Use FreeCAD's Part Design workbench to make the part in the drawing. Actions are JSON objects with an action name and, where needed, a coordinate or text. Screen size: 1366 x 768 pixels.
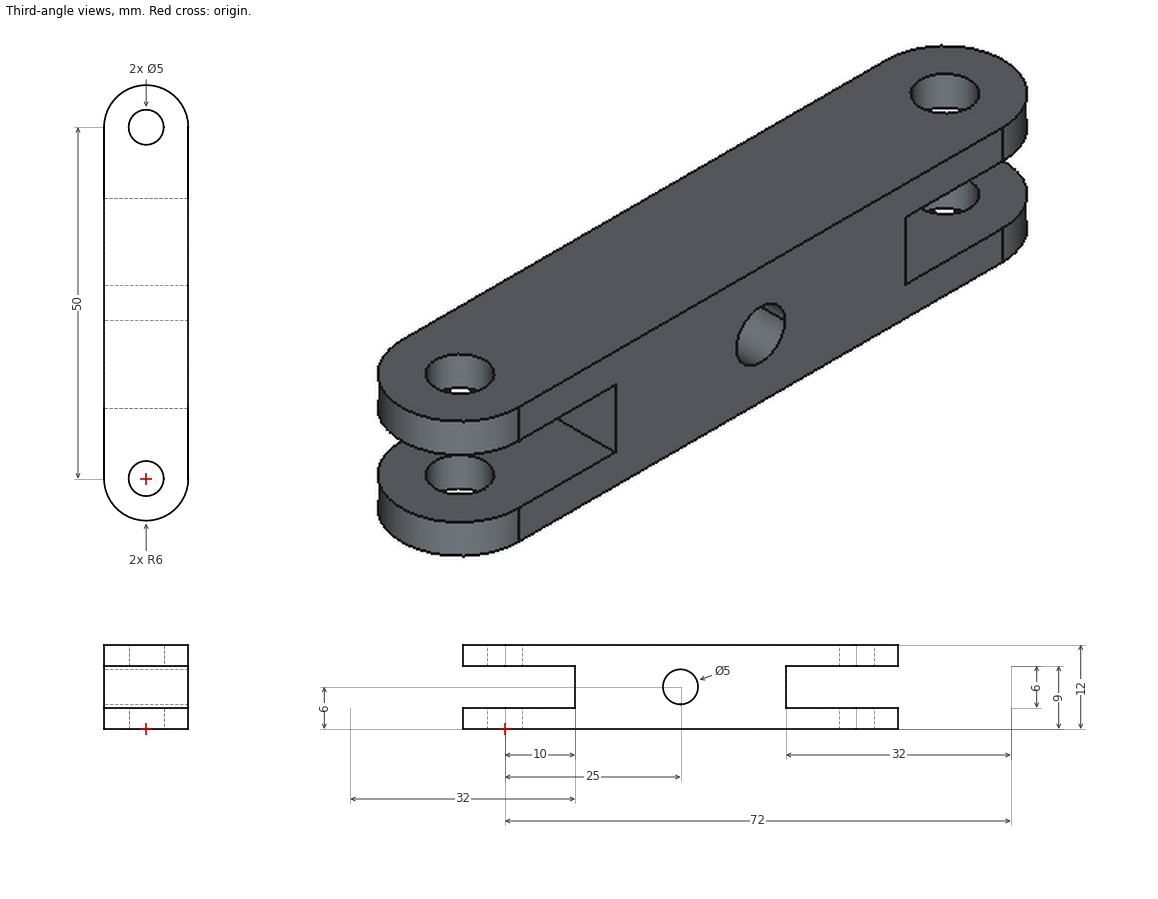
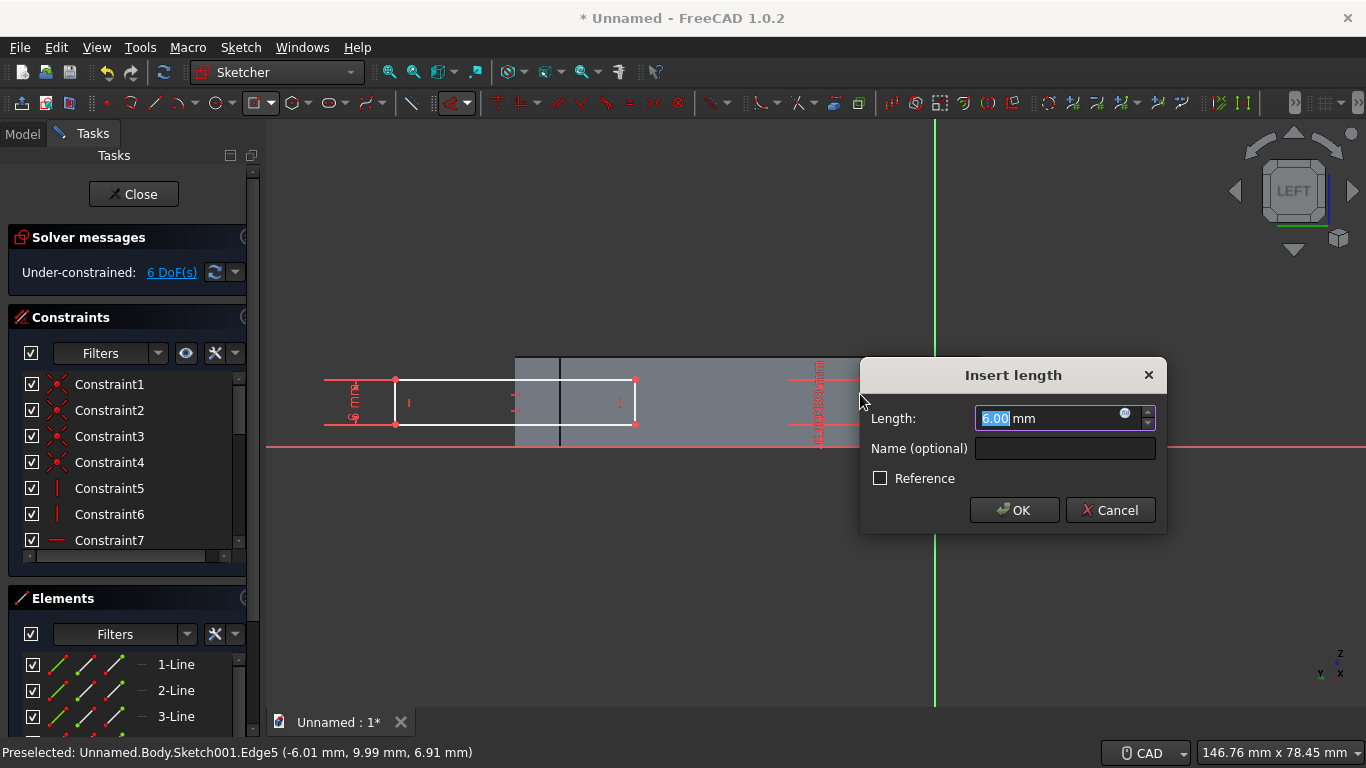
{"action": "type", "text": "6"}
{"action": "key", "text": "Return"}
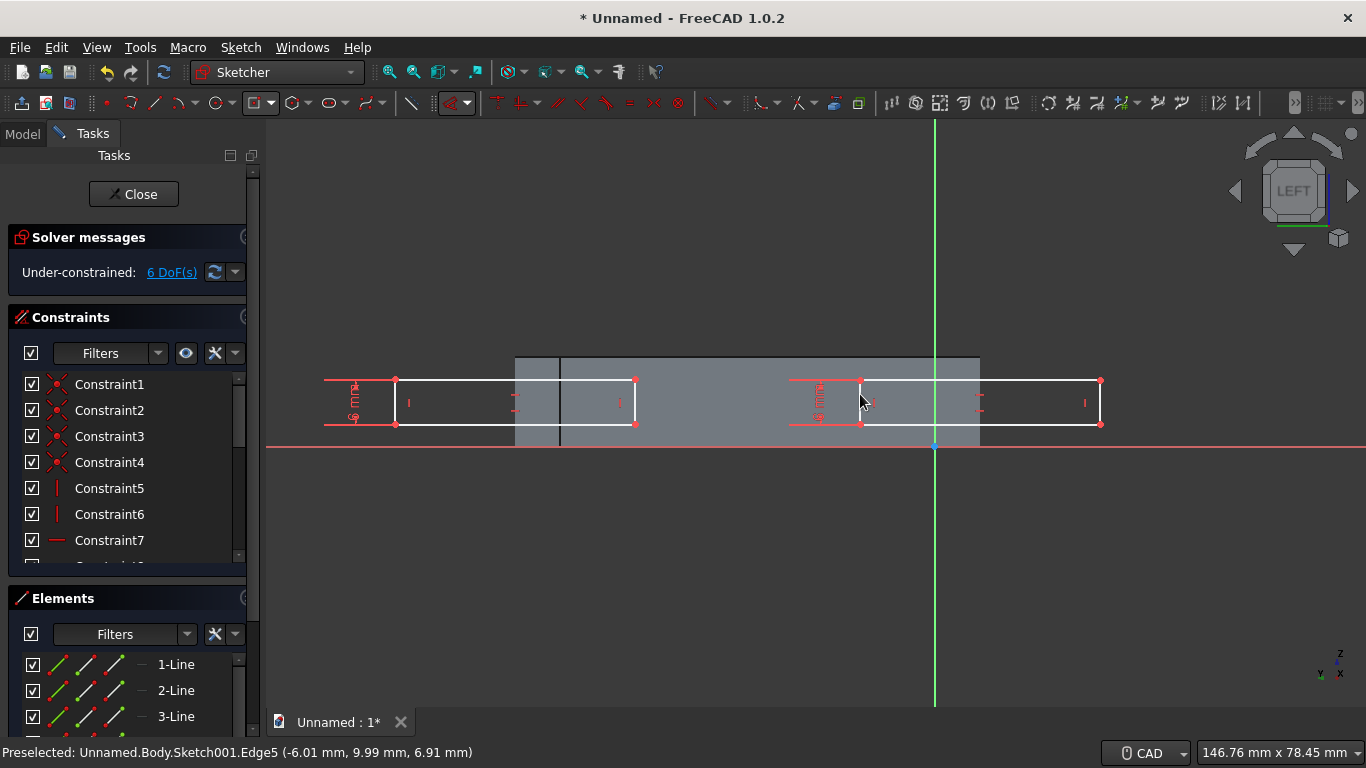
{"action": "left_click", "coordinate": [467, 425]}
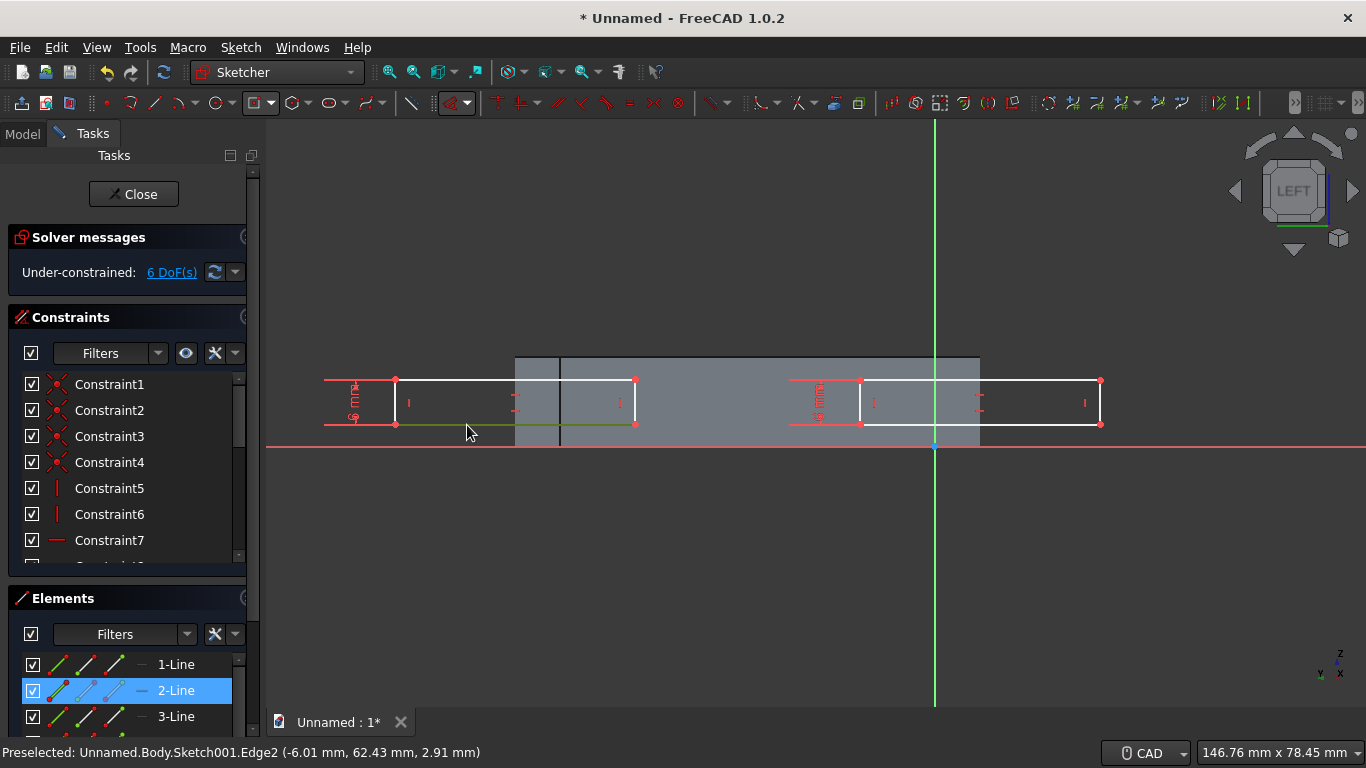
{"action": "key", "text": "l"}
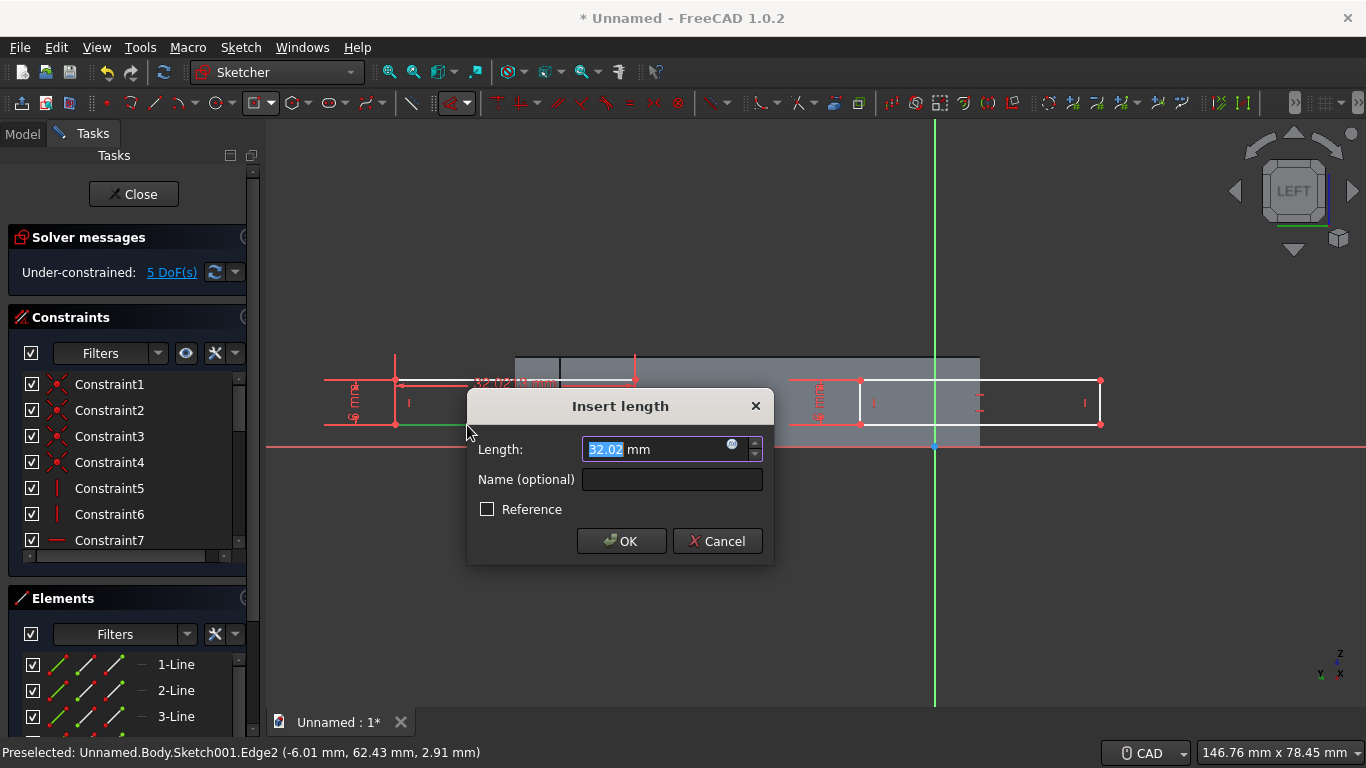
{"action": "type", "text": "32"}
{"action": "key", "text": "Return"}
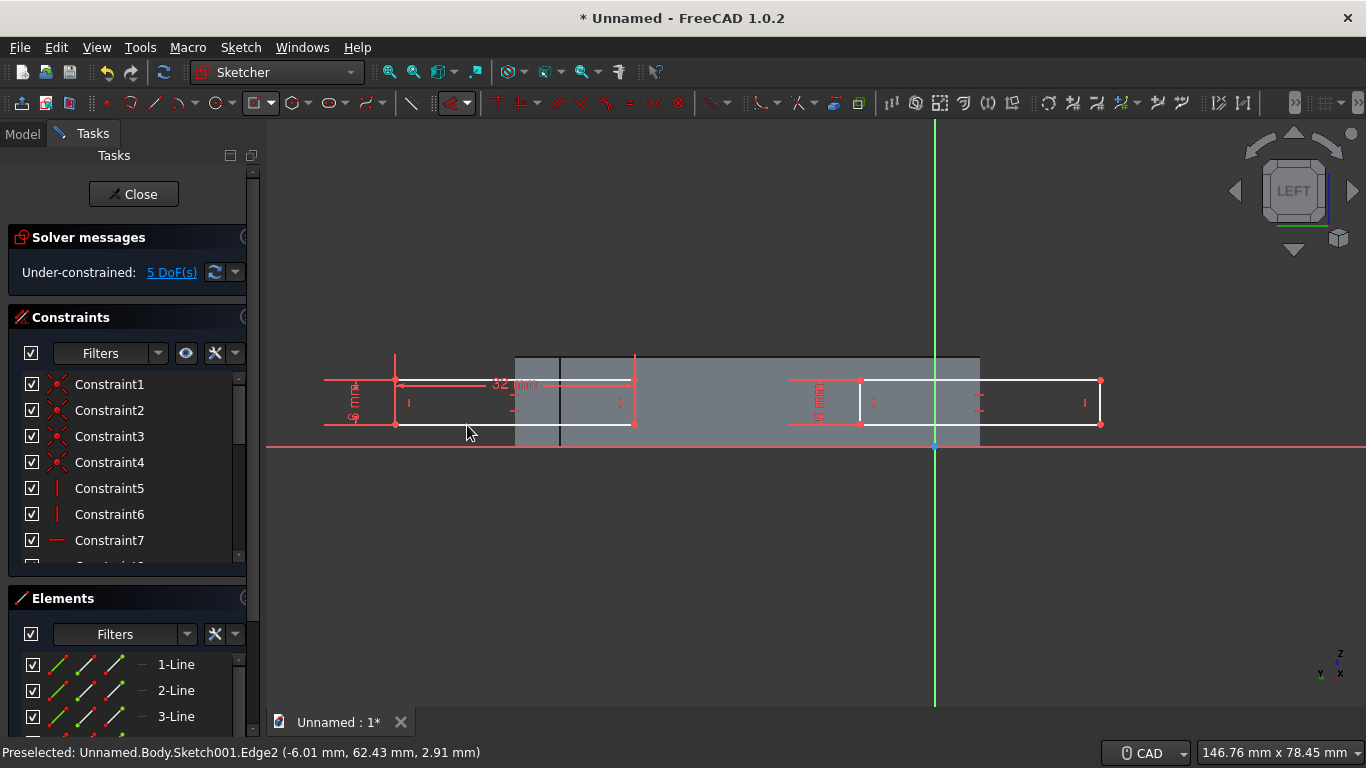
{"action": "left_click", "coordinate": [932, 425]}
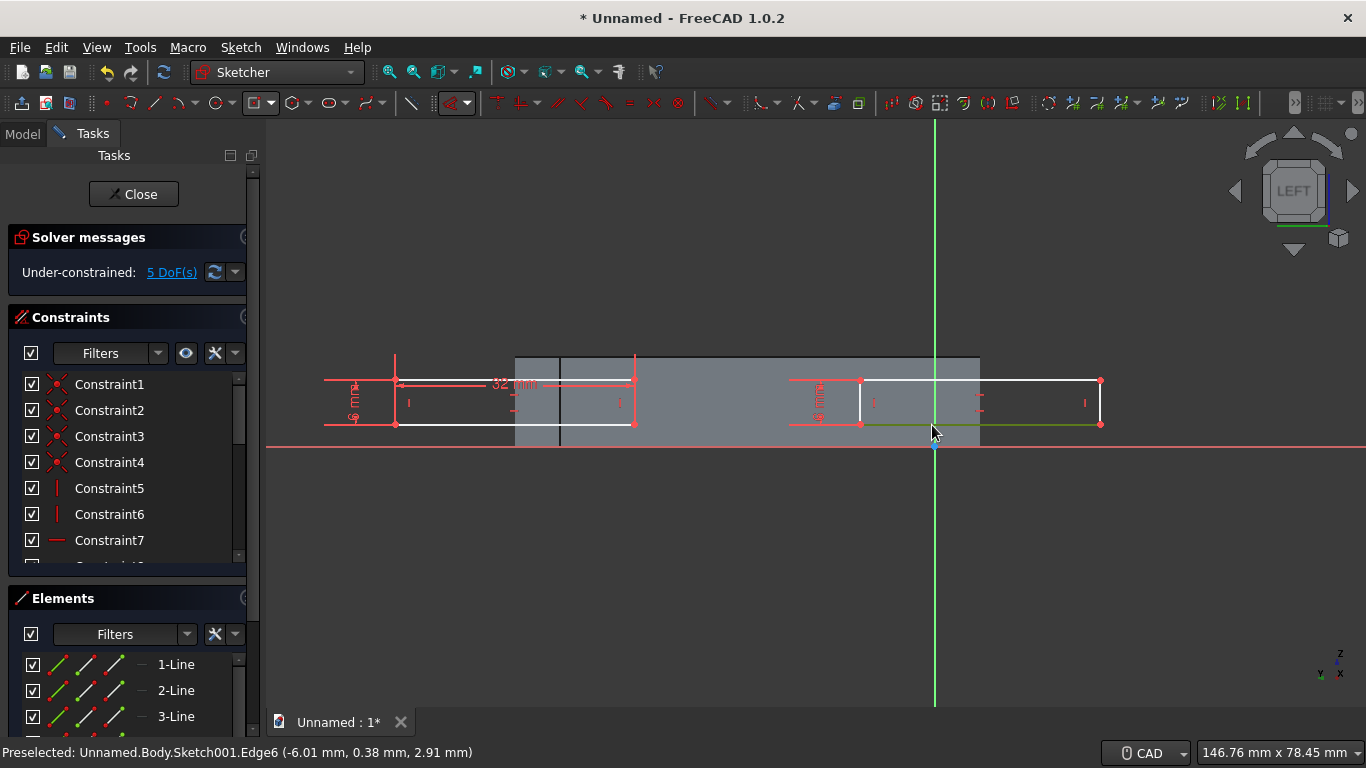
{"action": "key", "text": "l"}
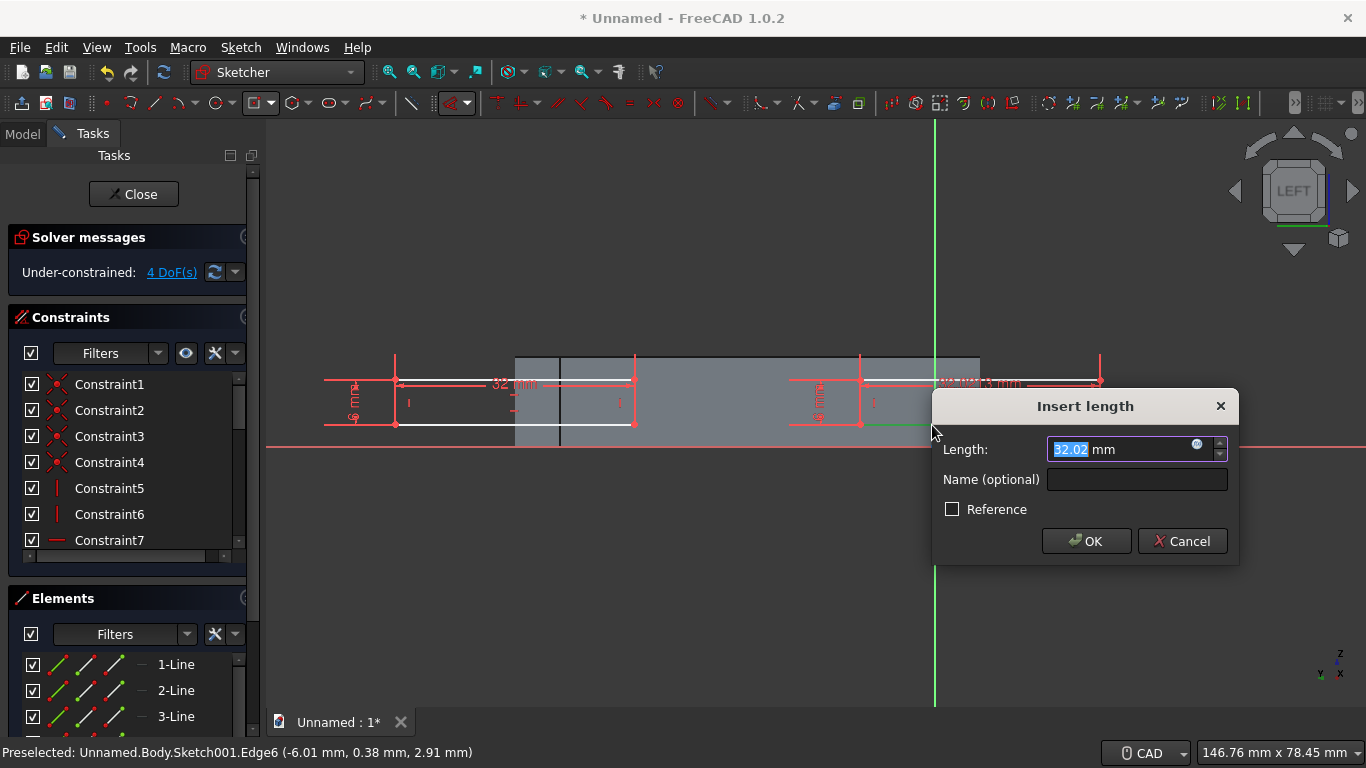
{"action": "type", "text": "32"}
{"action": "key", "text": "Return"}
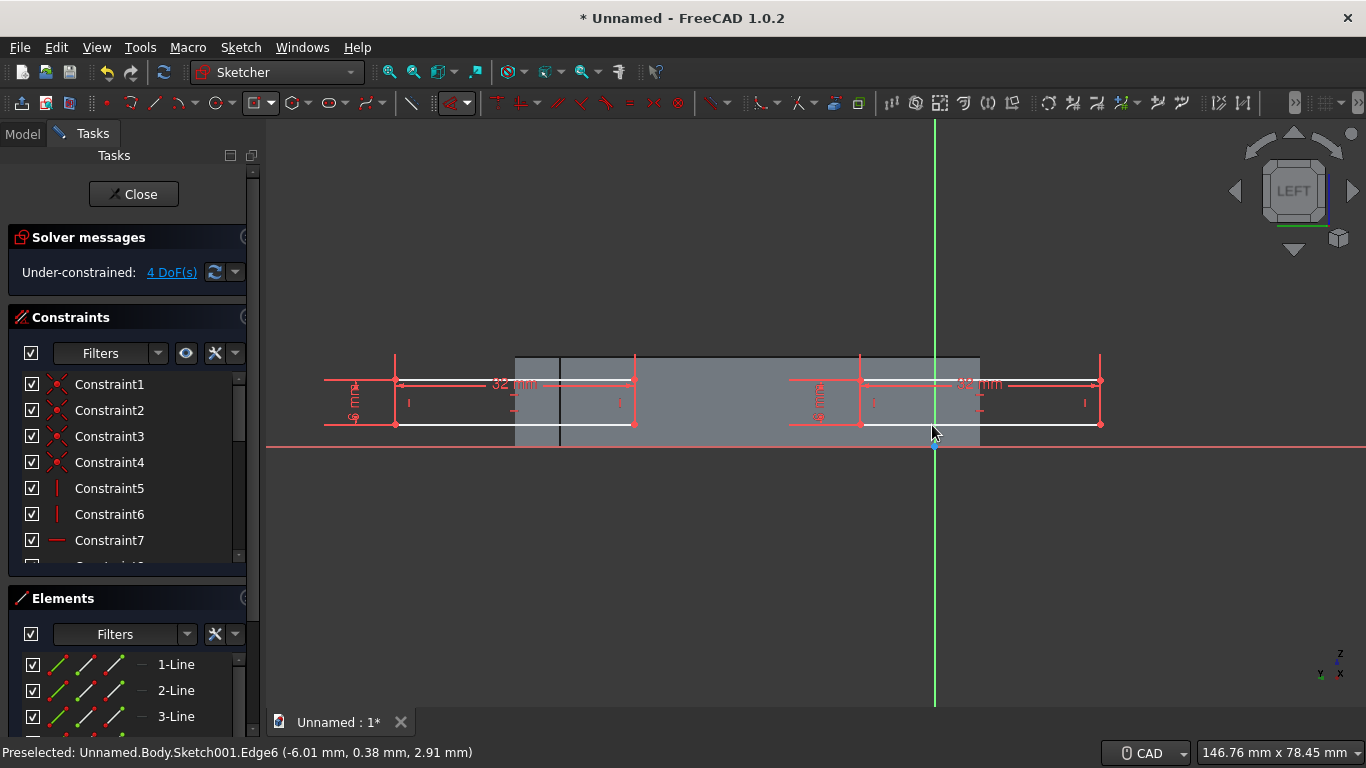
{"action": "left_click", "coordinate": [395, 380]}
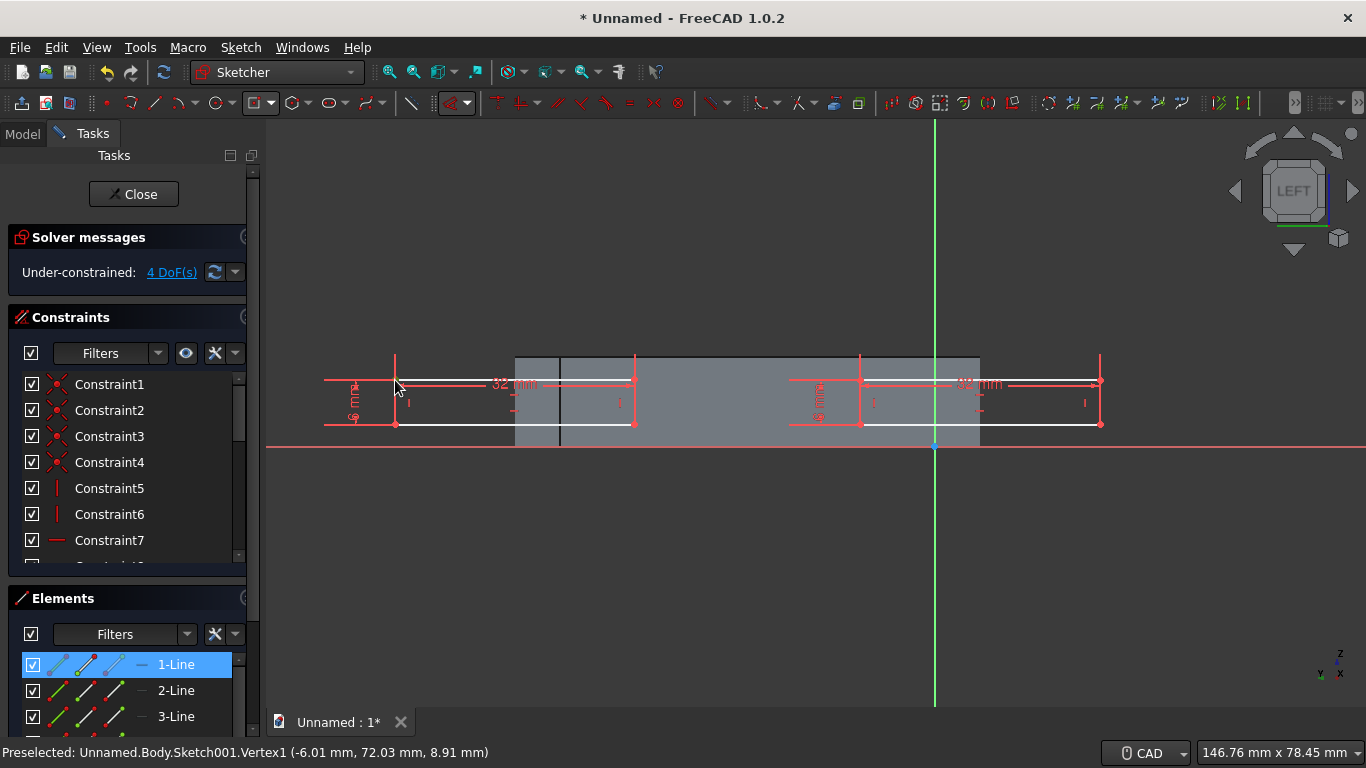
{"action": "key", "text": "i"}